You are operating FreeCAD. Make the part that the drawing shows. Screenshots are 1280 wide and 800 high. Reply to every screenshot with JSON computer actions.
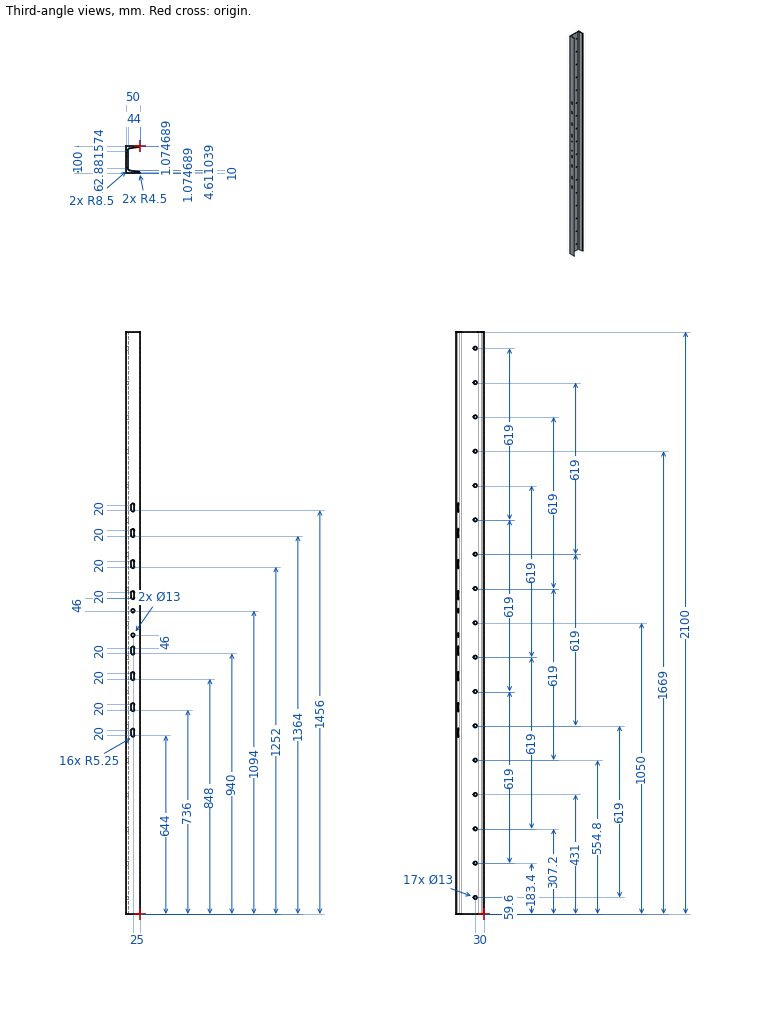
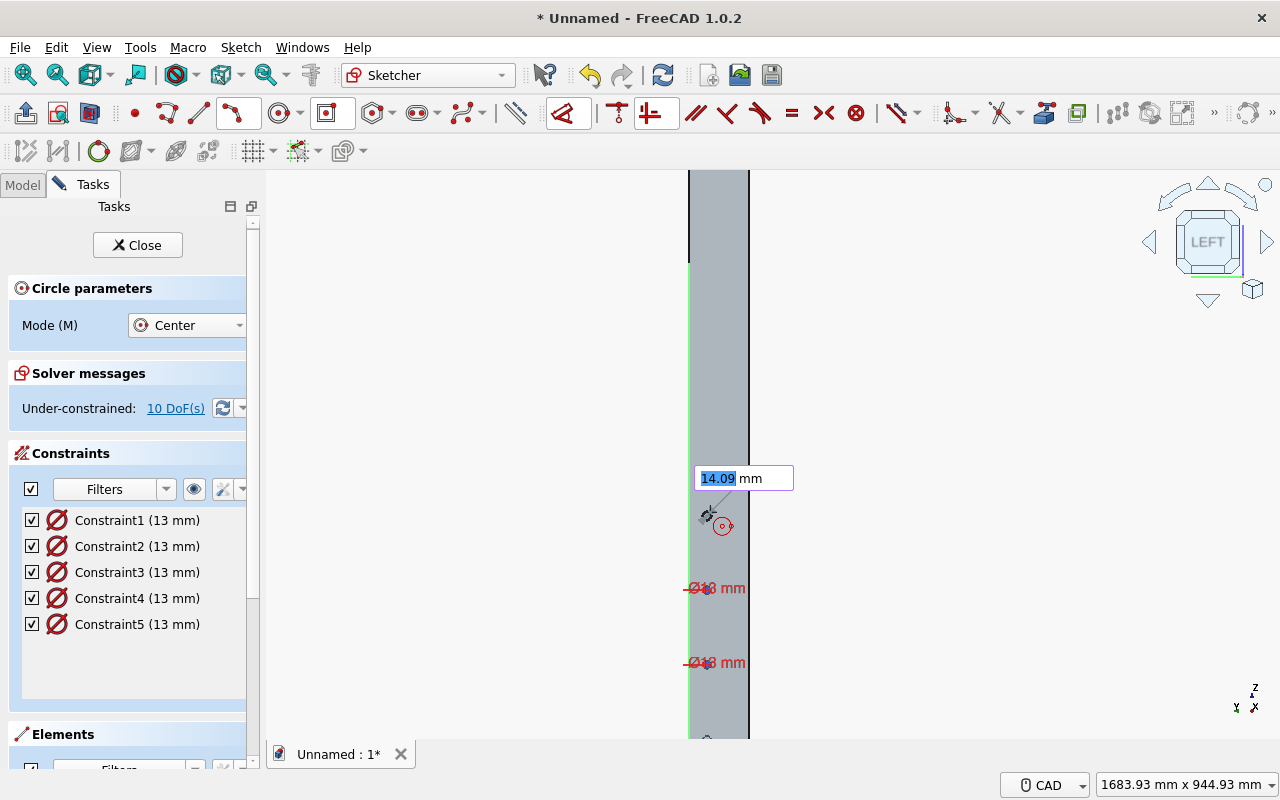
{"action": "type", "text": "13"}
{"action": "key", "text": "Return"}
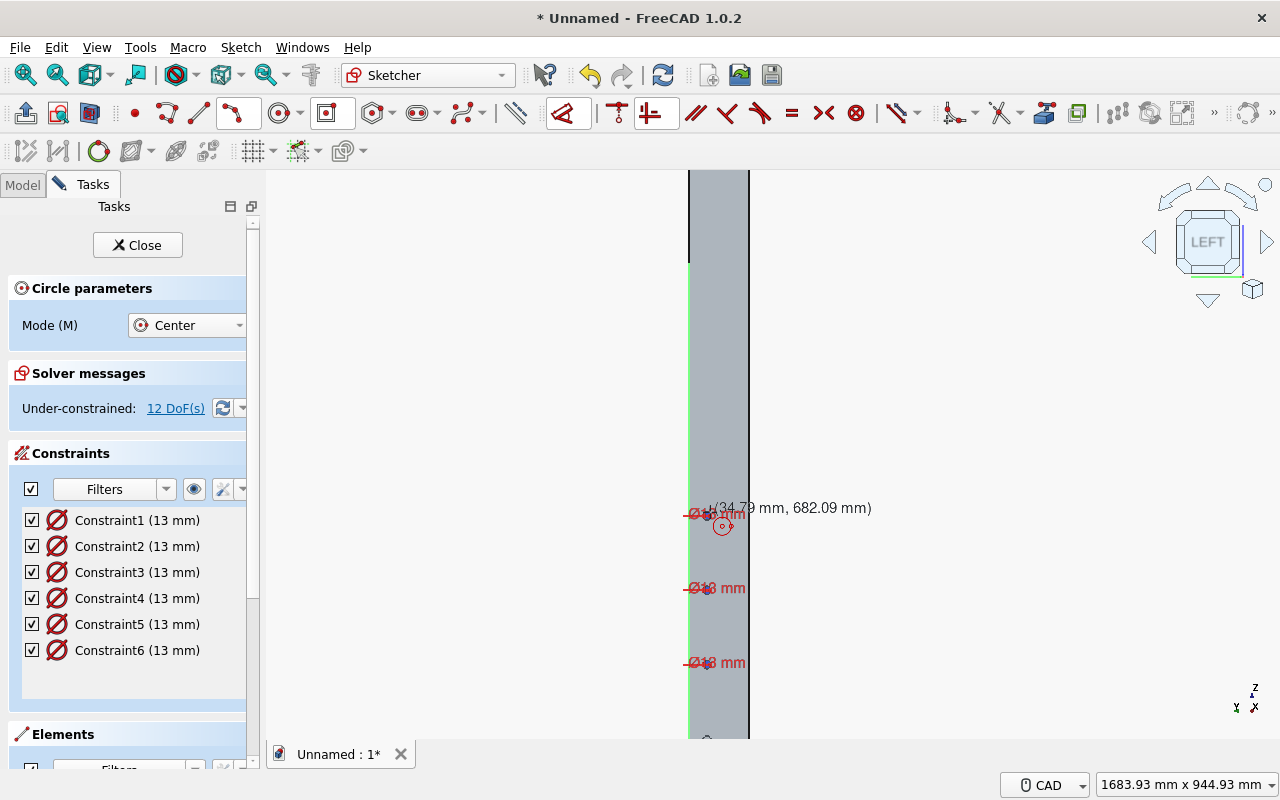
{"action": "scroll", "coordinate": [707, 441], "scroll_direction": "up", "scroll_amount": 9}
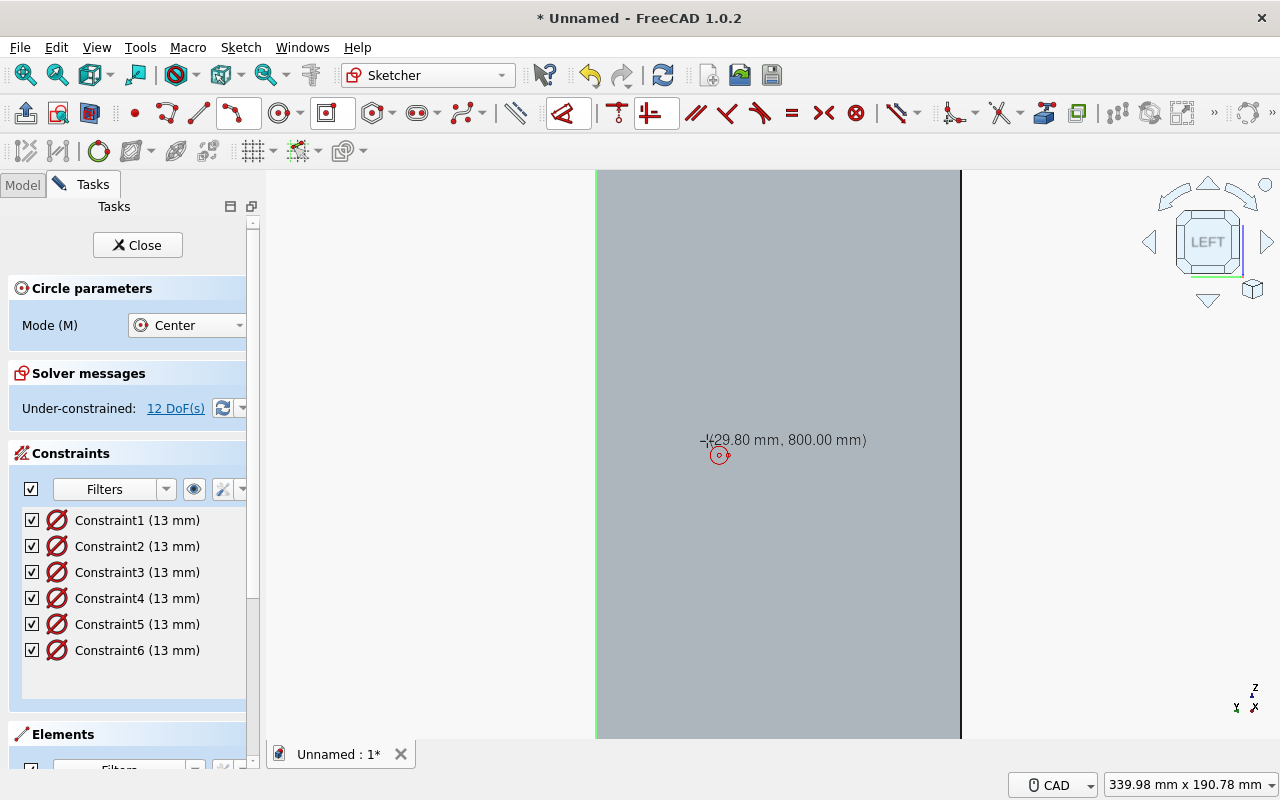
{"action": "scroll", "coordinate": [707, 498], "scroll_direction": "down", "scroll_amount": 15}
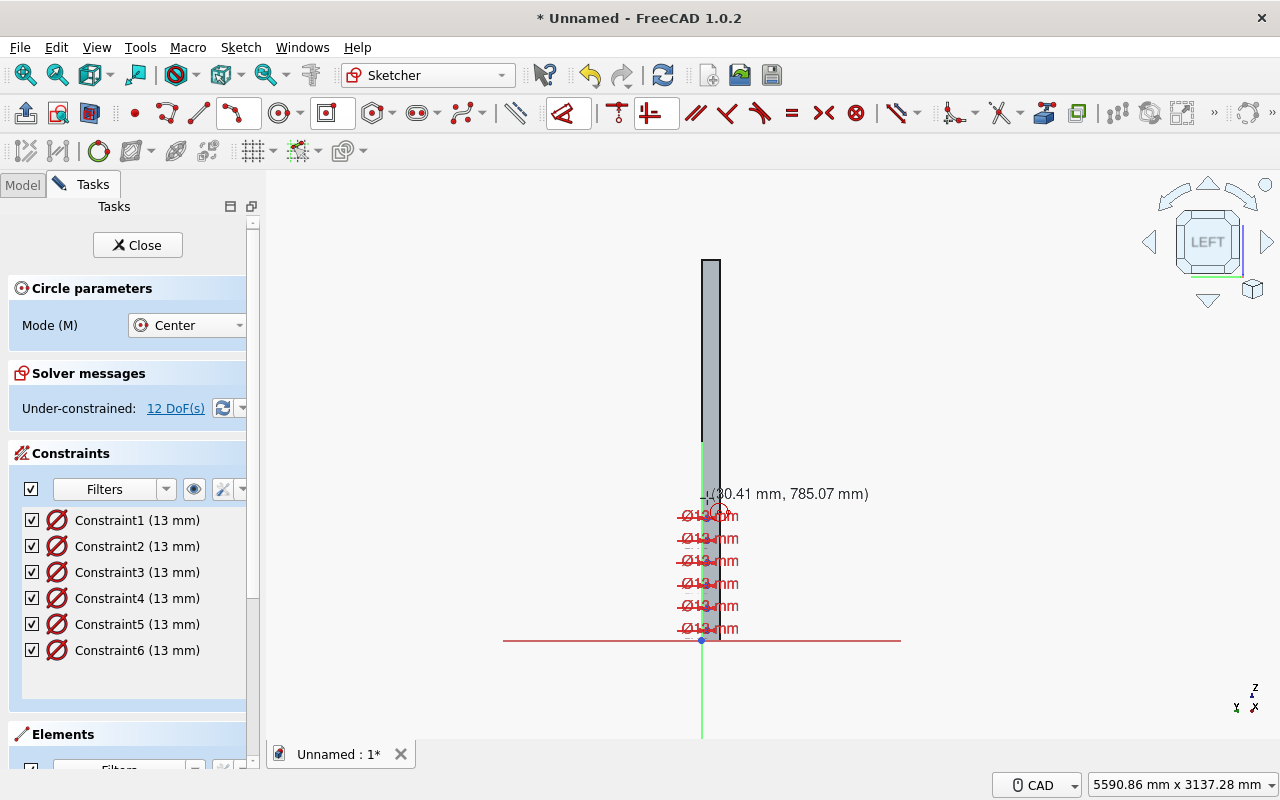
{"action": "scroll", "coordinate": [707, 495], "scroll_direction": "up", "scroll_amount": 6}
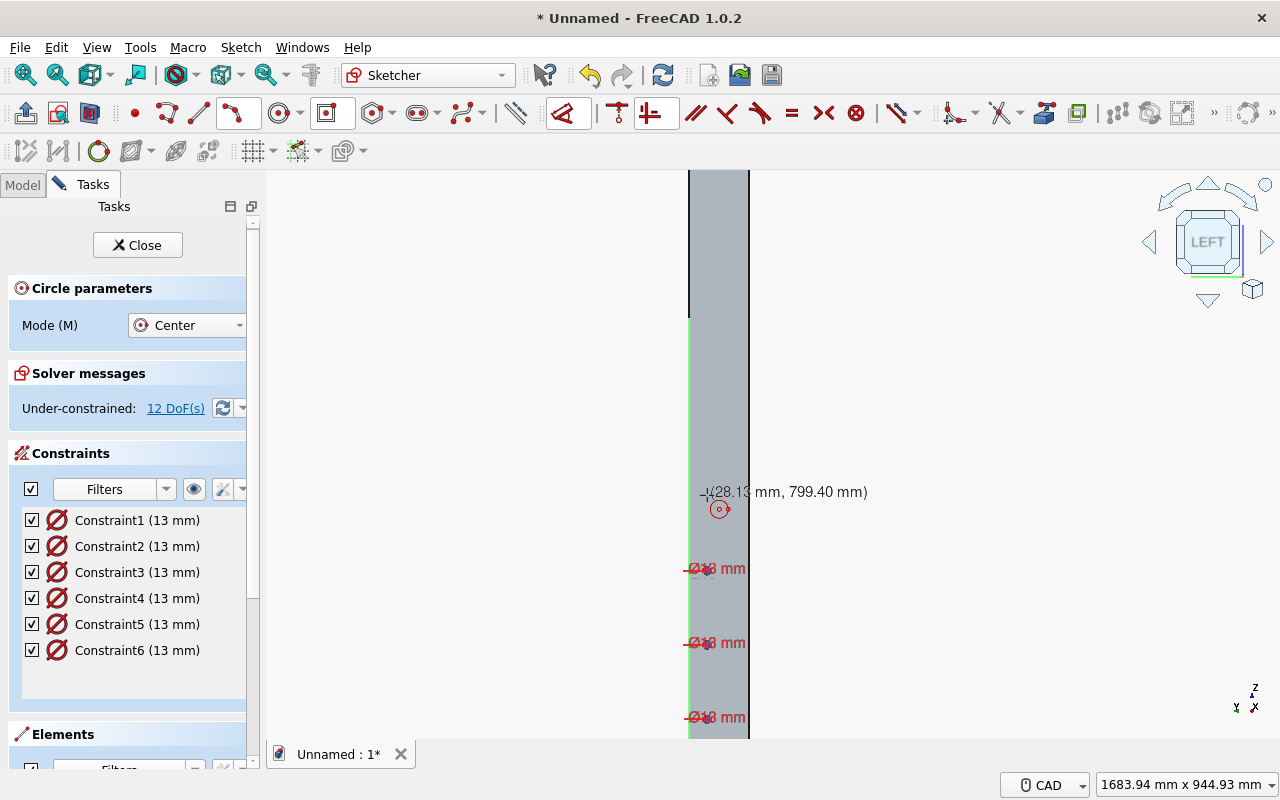
{"action": "left_click", "coordinate": [707, 495]}
{"action": "mouse_move", "coordinate": [710, 492]}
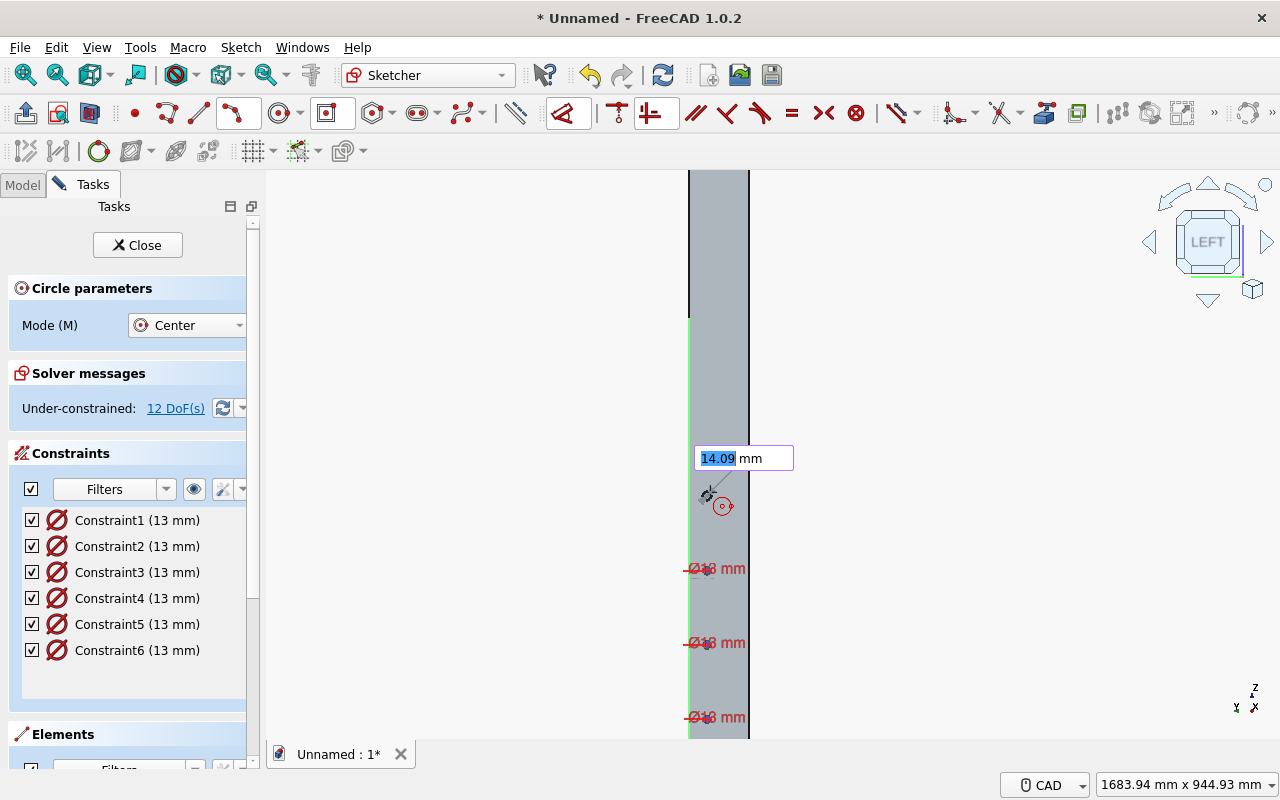
{"action": "type", "text": "13"}
{"action": "key", "text": "Return"}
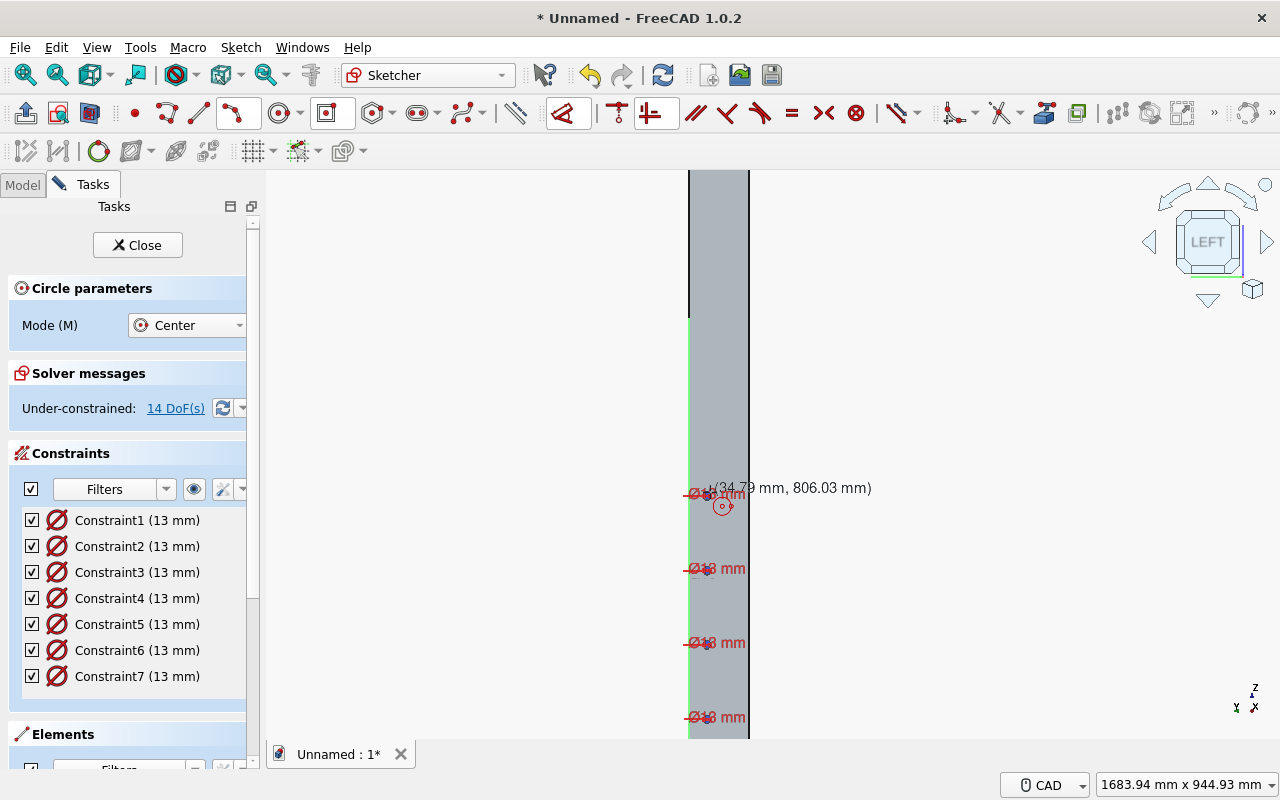
{"action": "scroll", "coordinate": [707, 421], "scroll_direction": "up", "scroll_amount": 9}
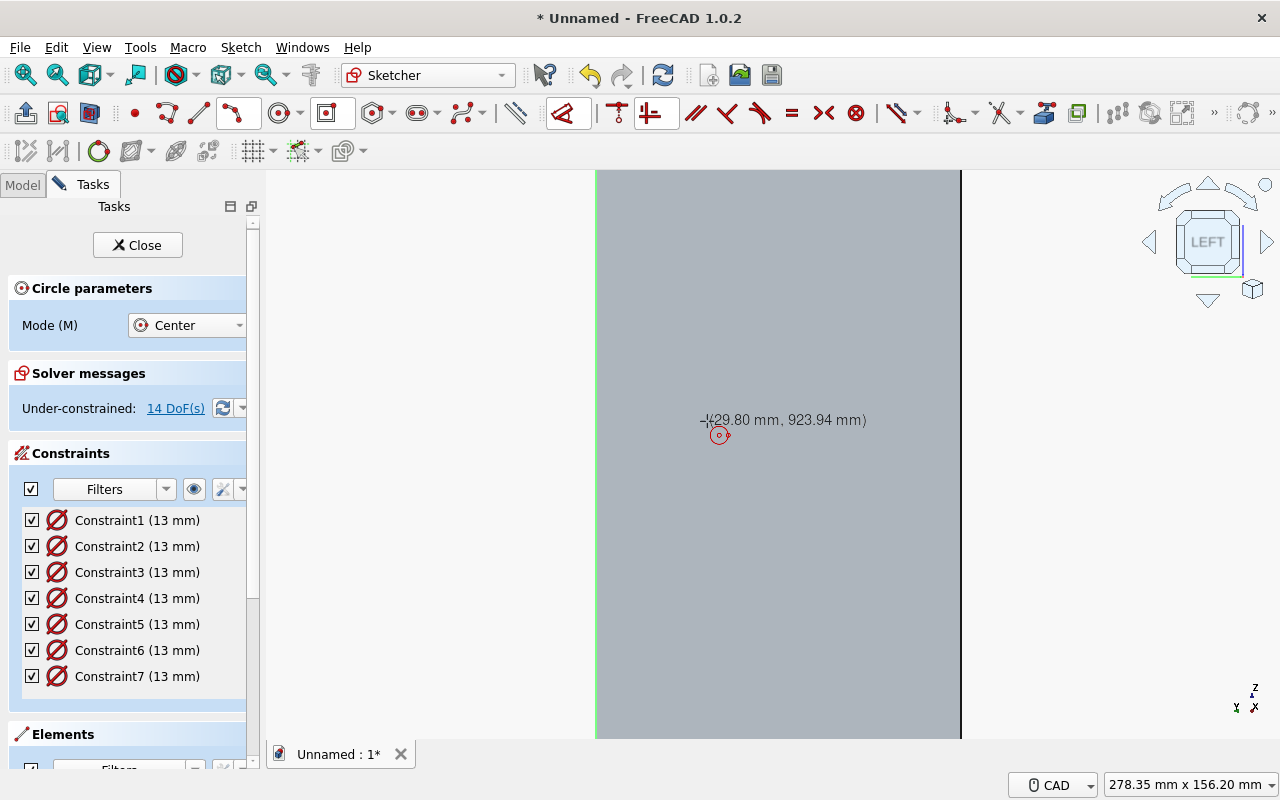
{"action": "scroll", "coordinate": [707, 475], "scroll_direction": "down", "scroll_amount": 15}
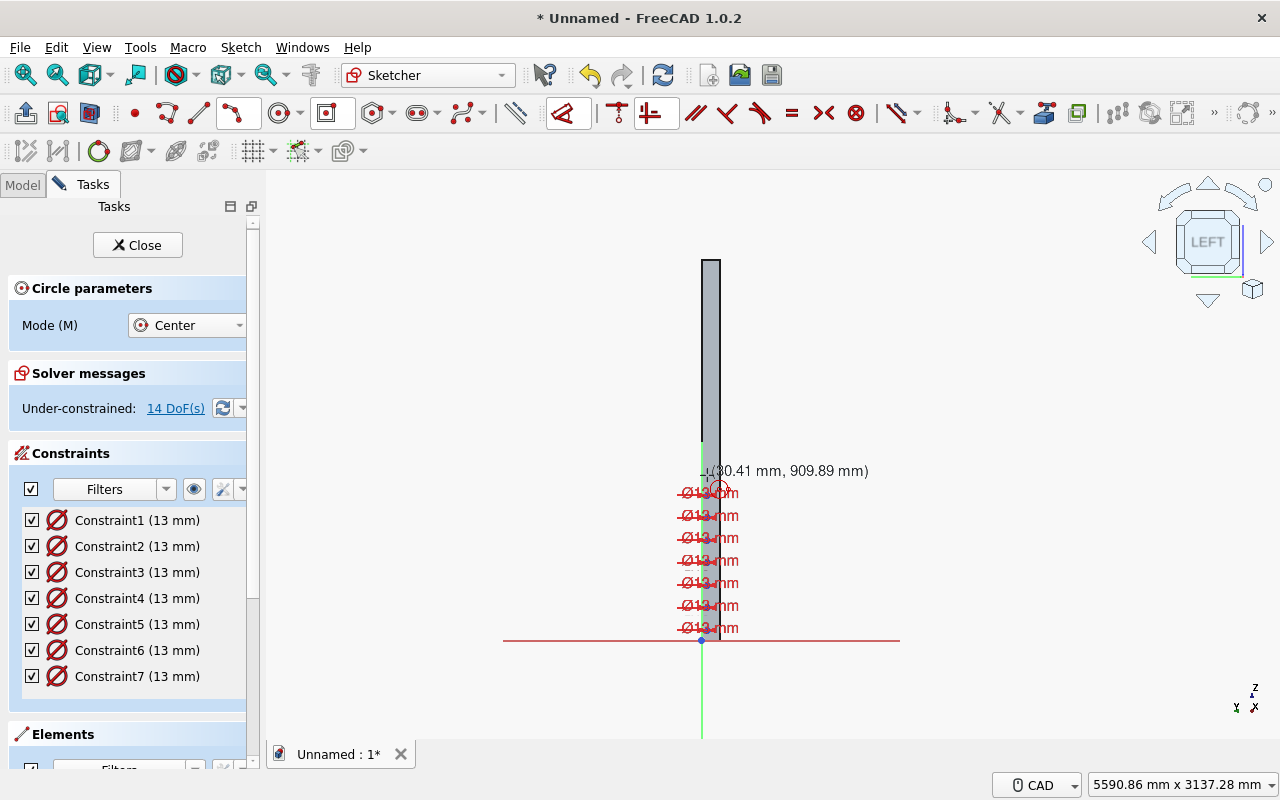
{"action": "scroll", "coordinate": [707, 473], "scroll_direction": "up", "scroll_amount": 6}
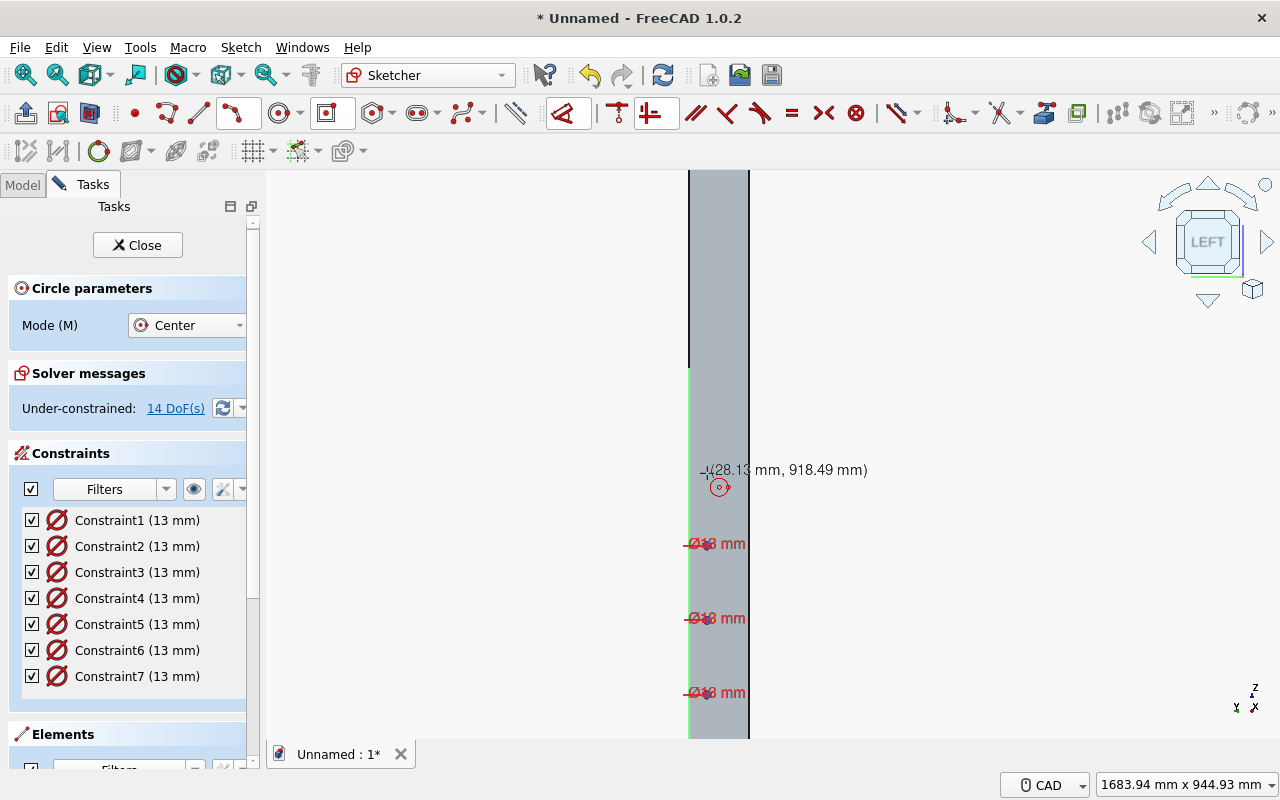
{"action": "left_click", "coordinate": [707, 470]}
{"action": "mouse_move", "coordinate": [710, 468]}